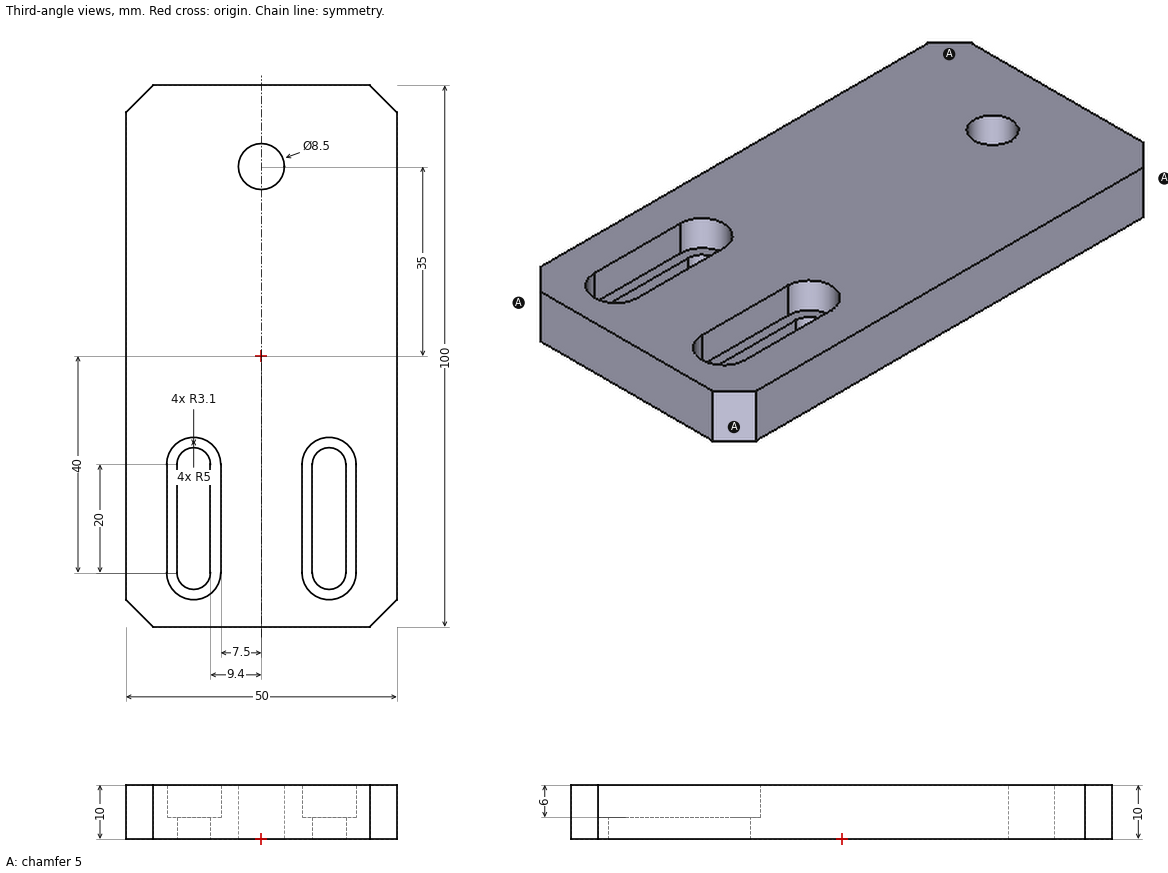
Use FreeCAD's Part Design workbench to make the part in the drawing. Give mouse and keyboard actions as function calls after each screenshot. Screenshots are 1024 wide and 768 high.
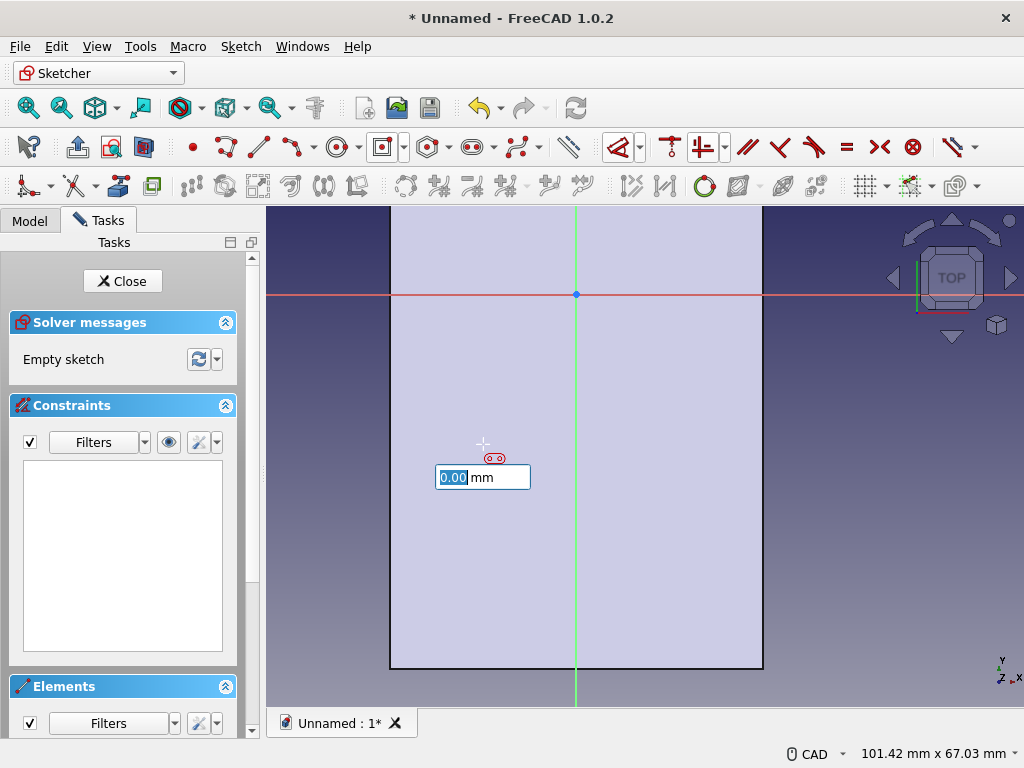
click(506, 519)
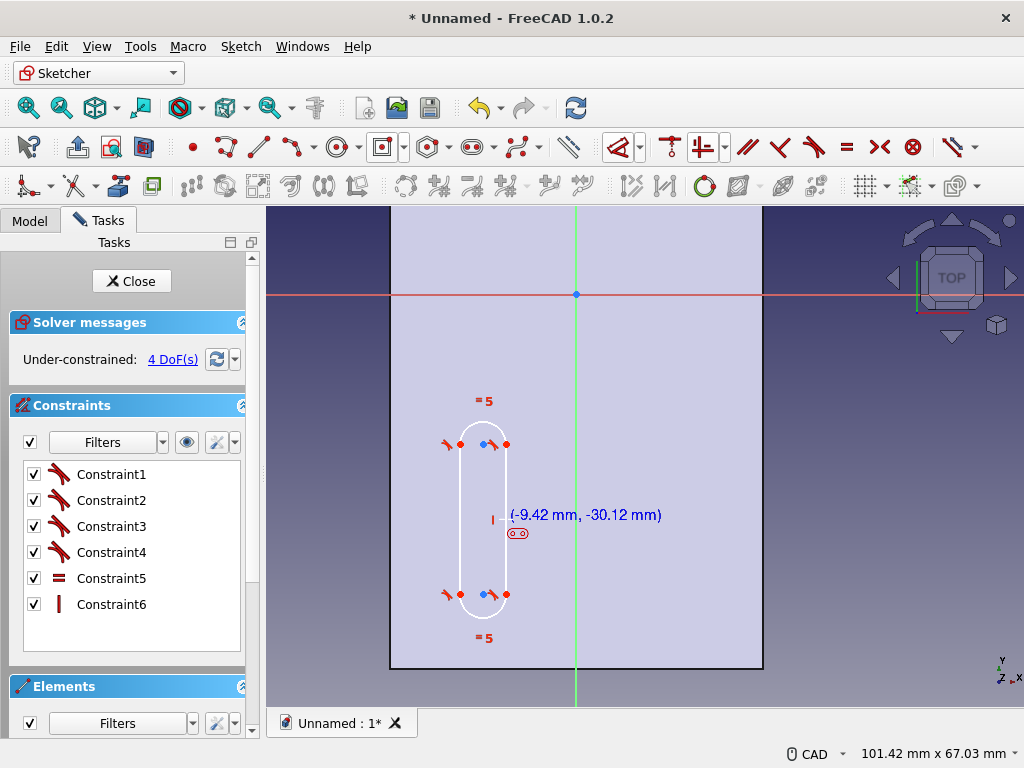
click(670, 594)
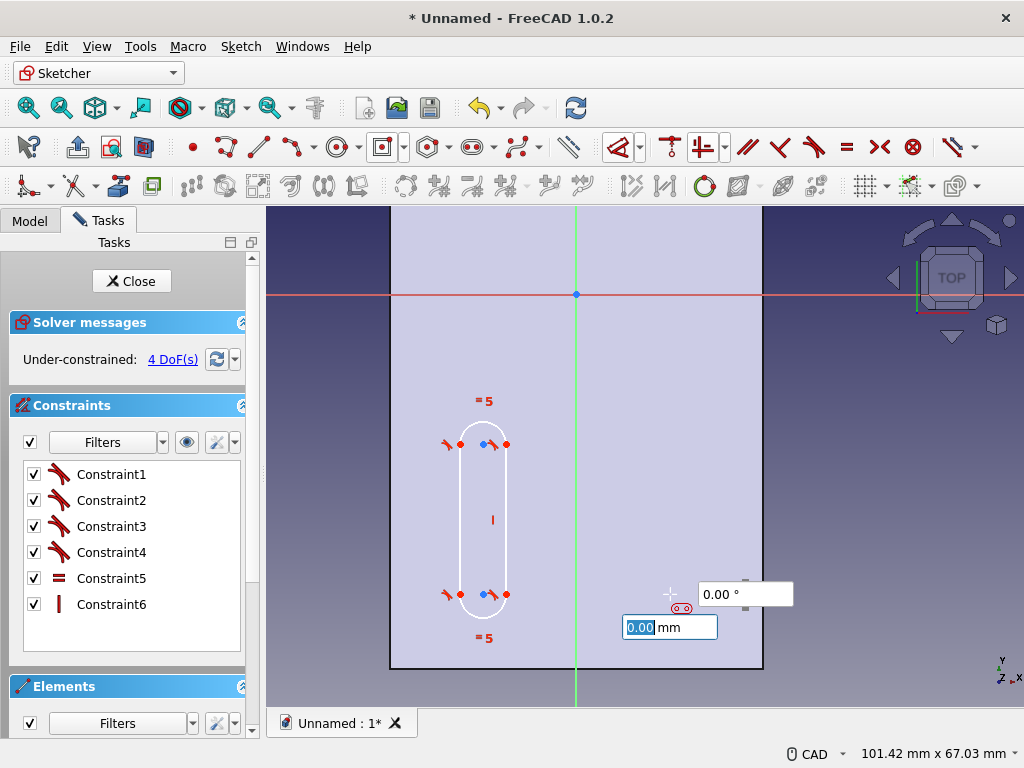
click(670, 444)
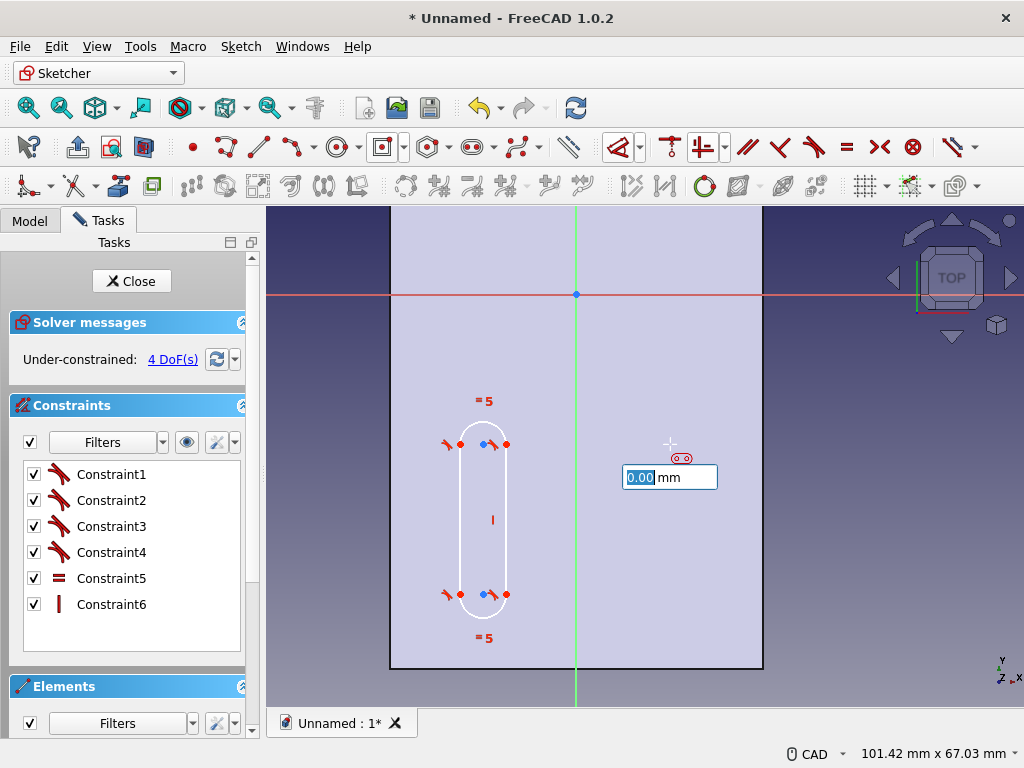
click(647, 519)
key(Escape)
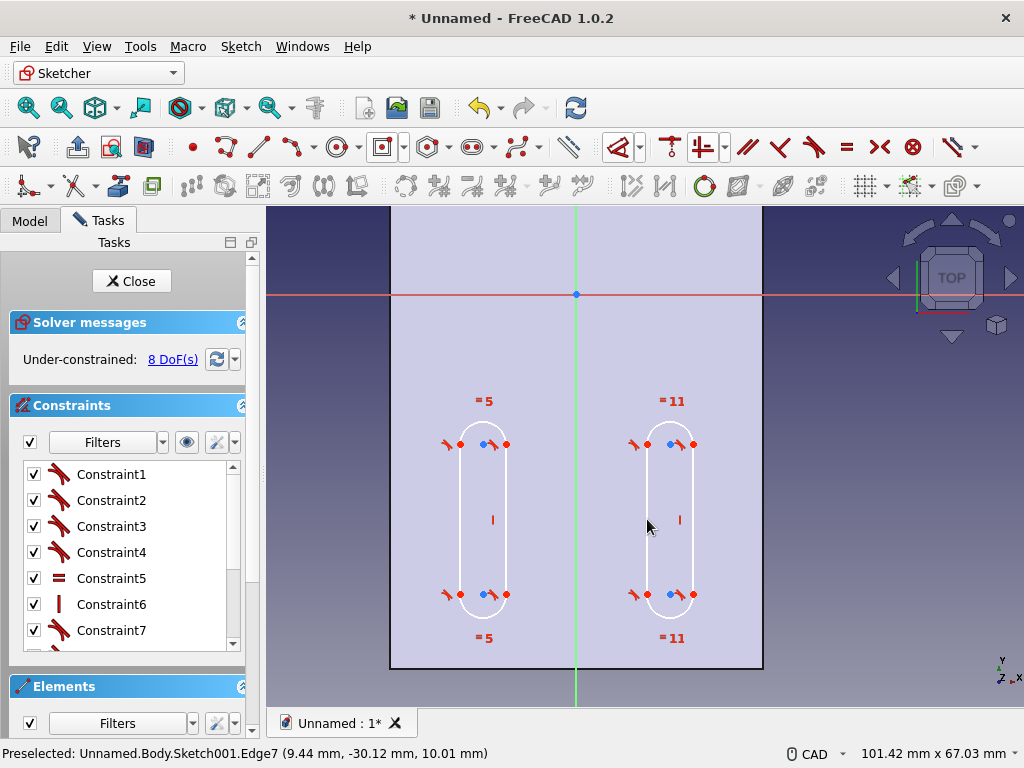
click(469, 614)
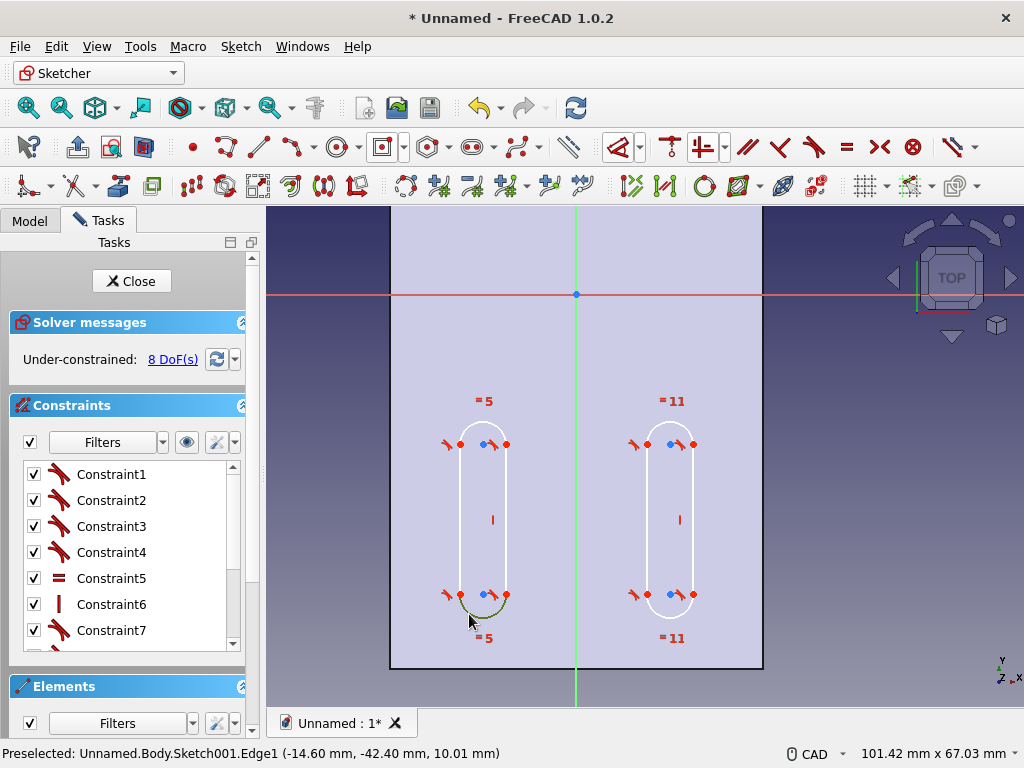
click(656, 614)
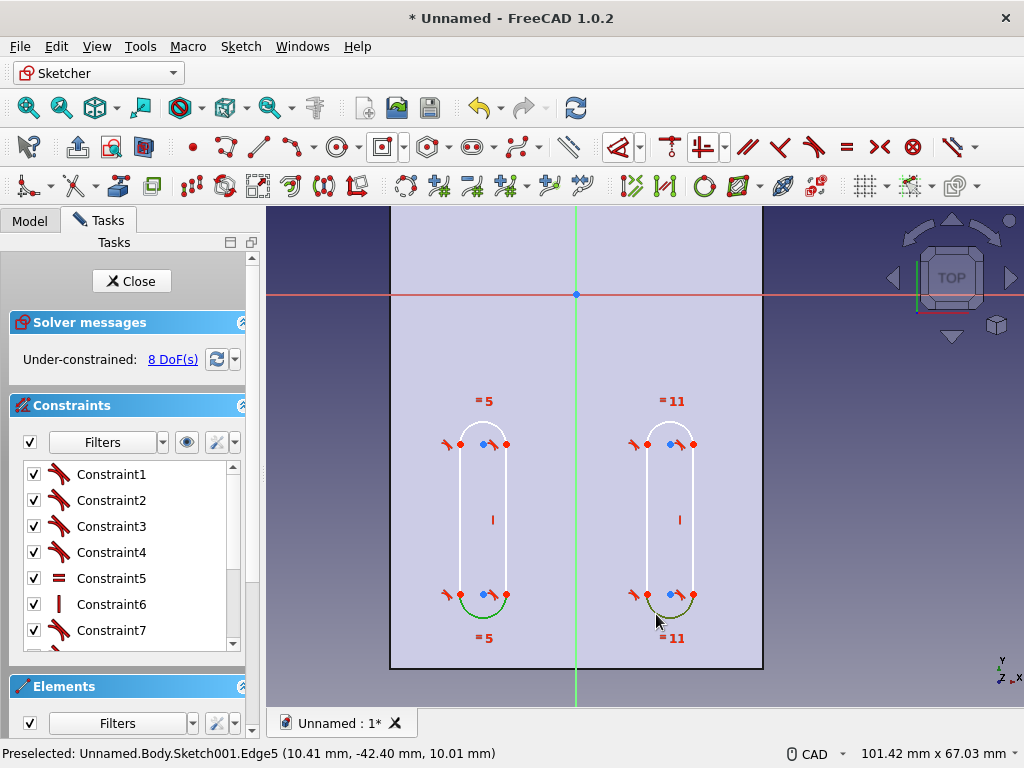
click(847, 148)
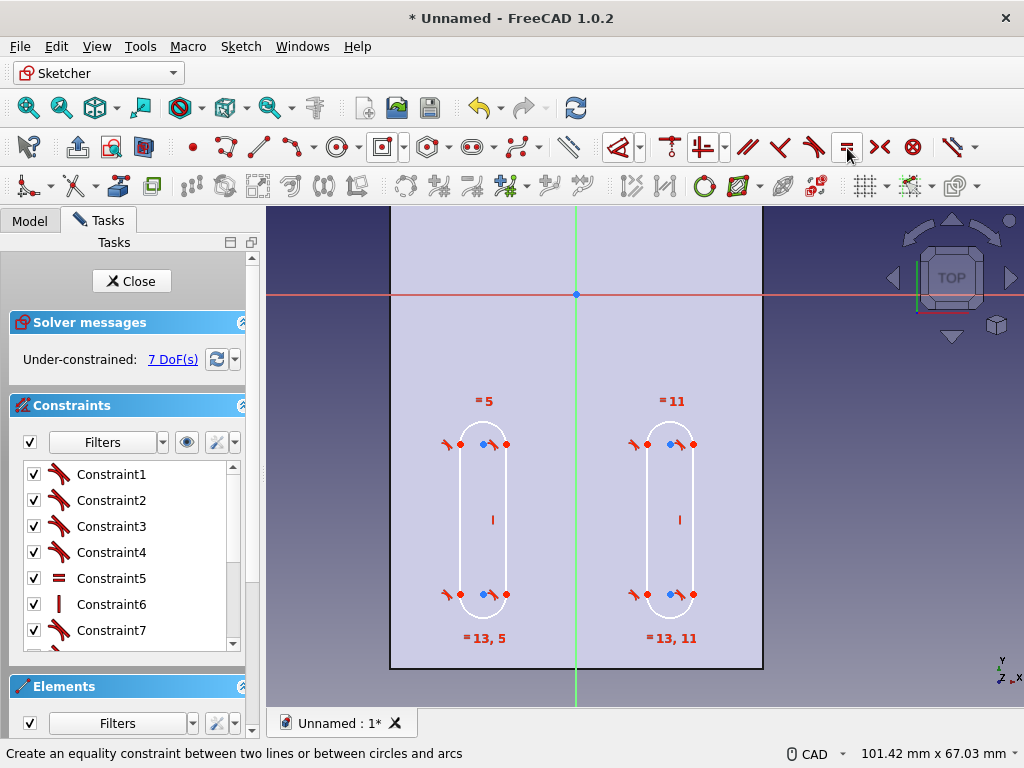
click(483, 595)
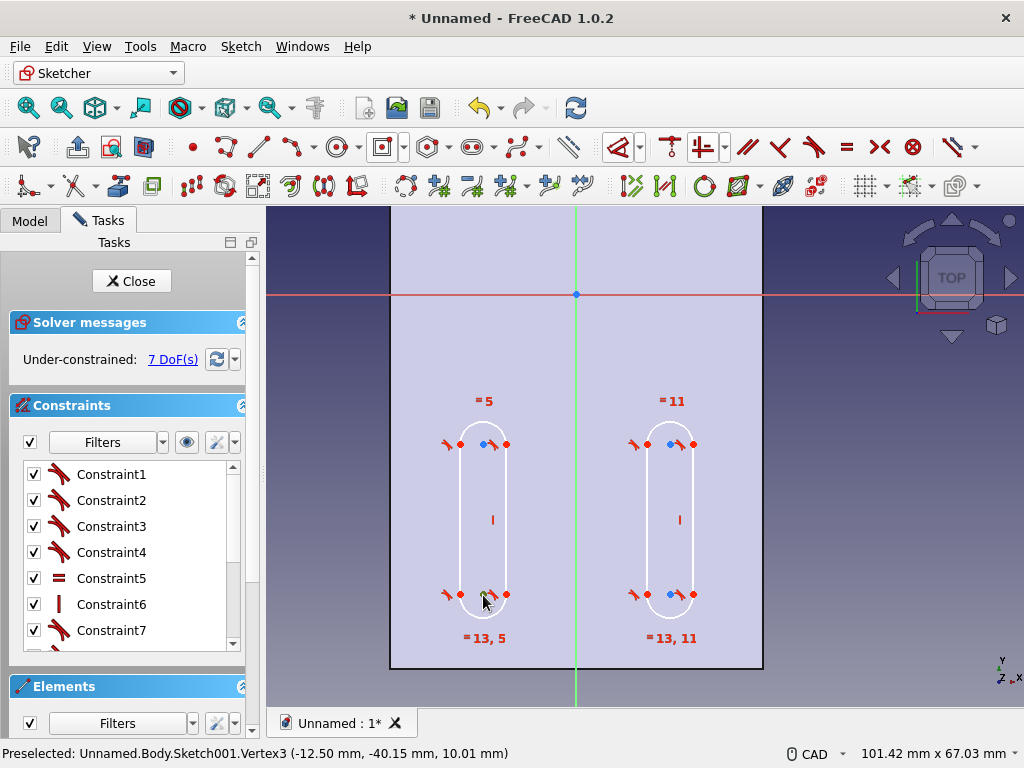
click(670, 595)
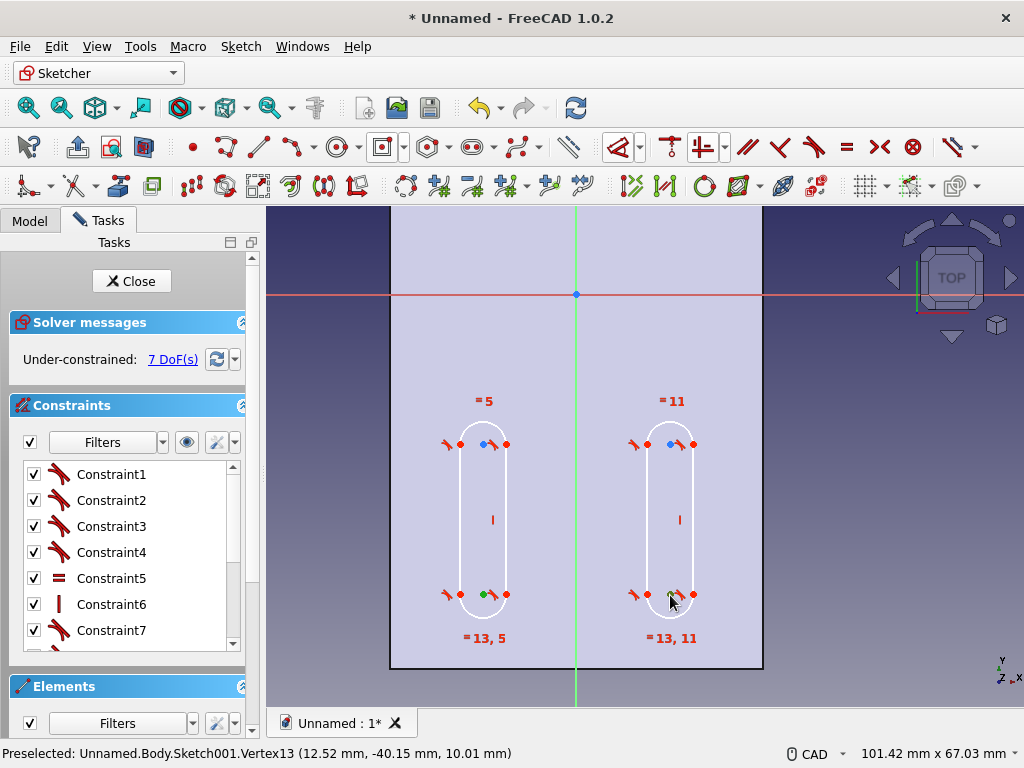
click(576, 647)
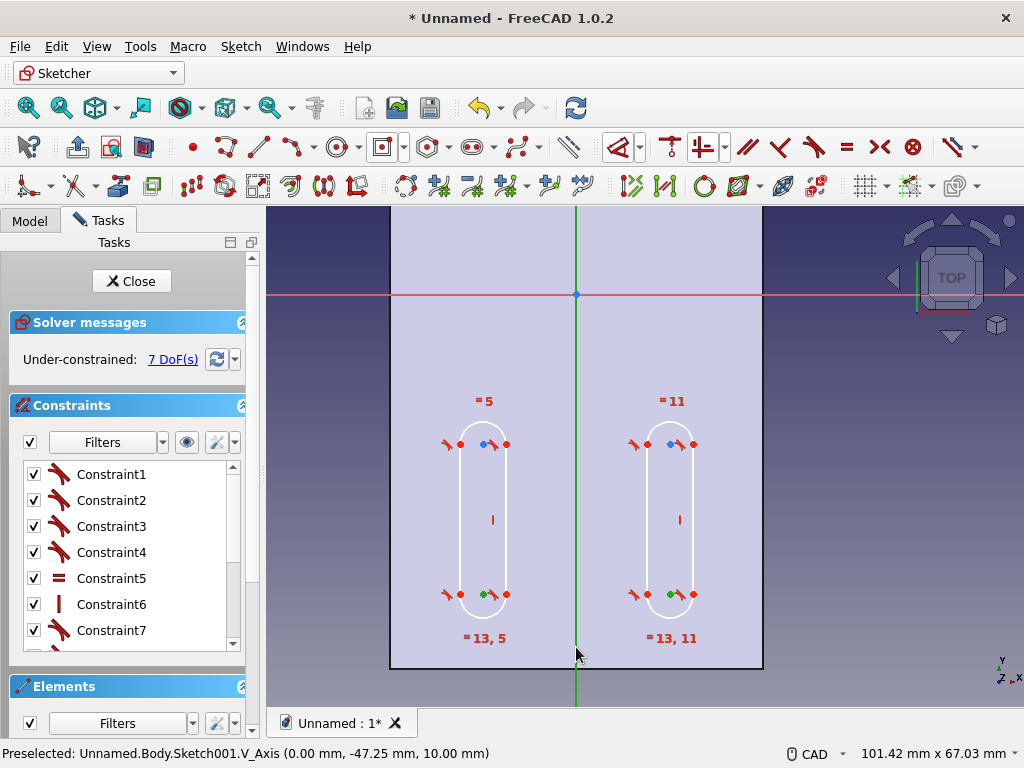
click(880, 148)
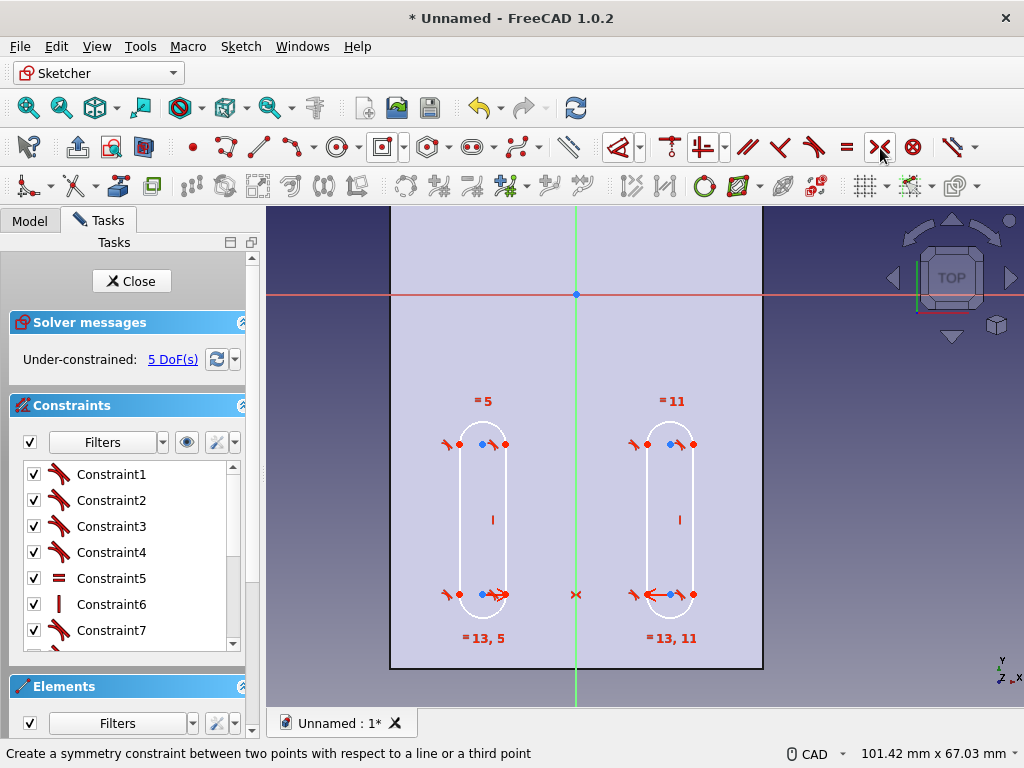
scroll(469, 614, up, 3)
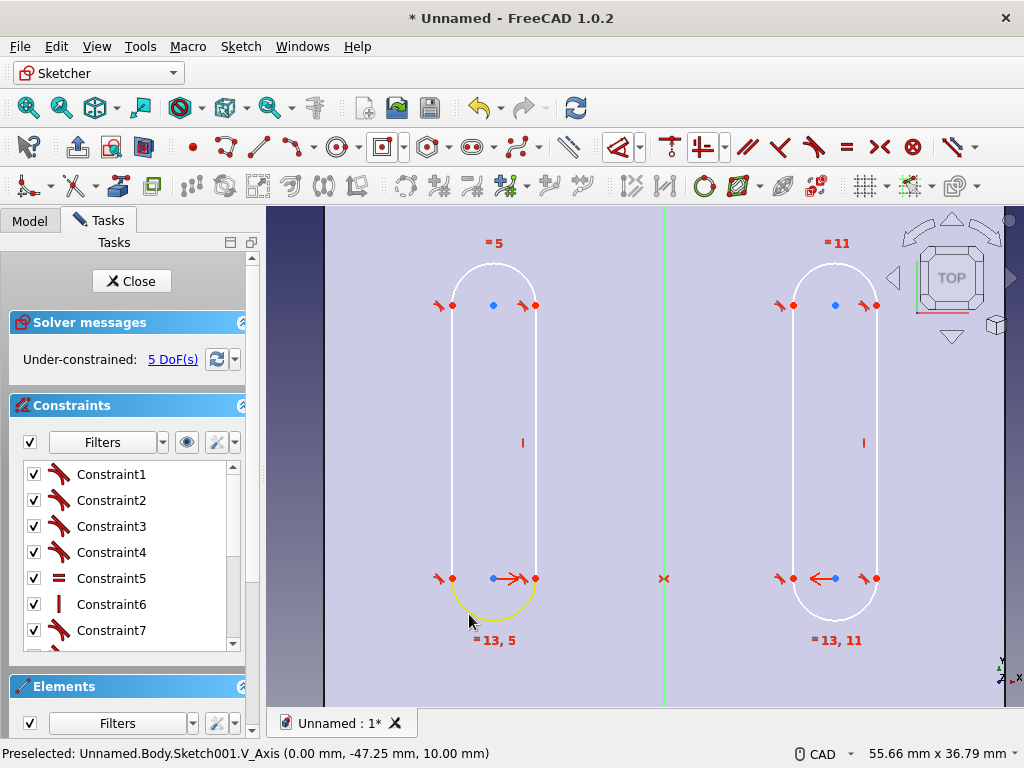
click(469, 613)